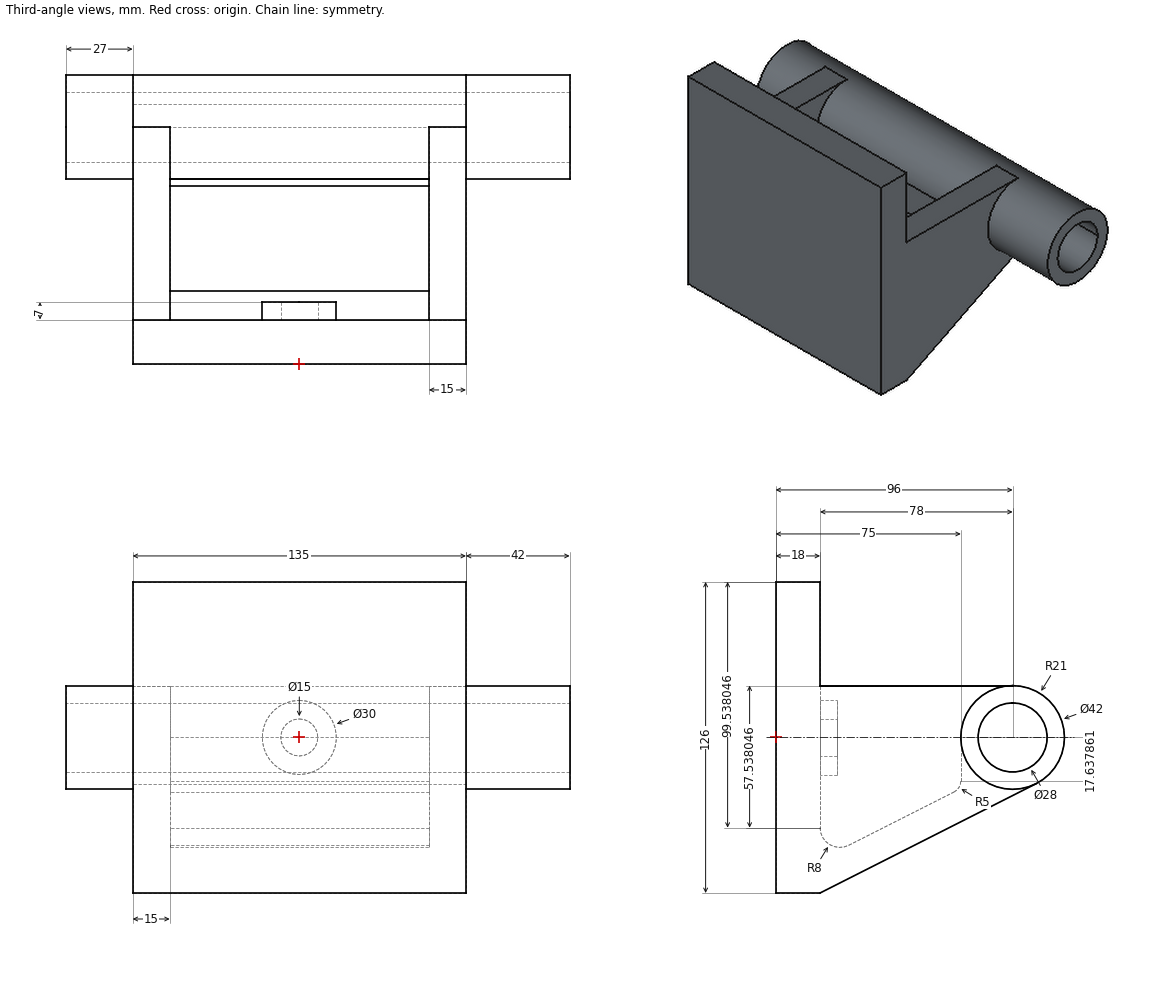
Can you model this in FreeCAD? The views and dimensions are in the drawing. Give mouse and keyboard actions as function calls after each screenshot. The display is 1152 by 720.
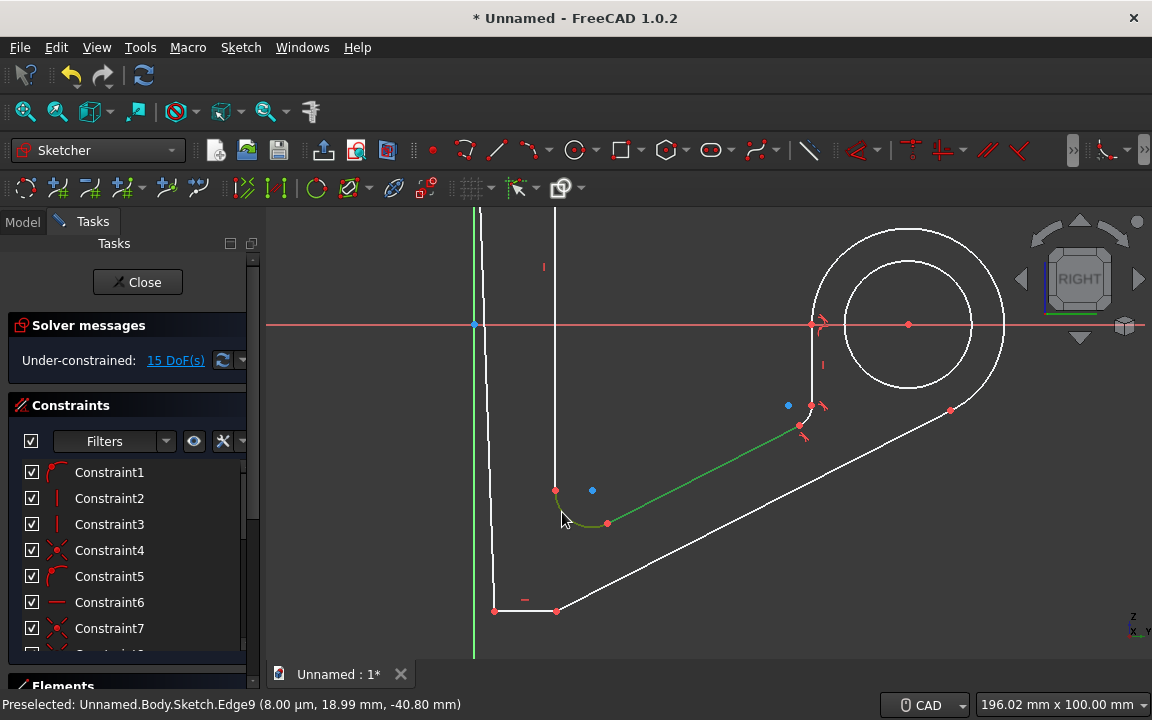
key(t)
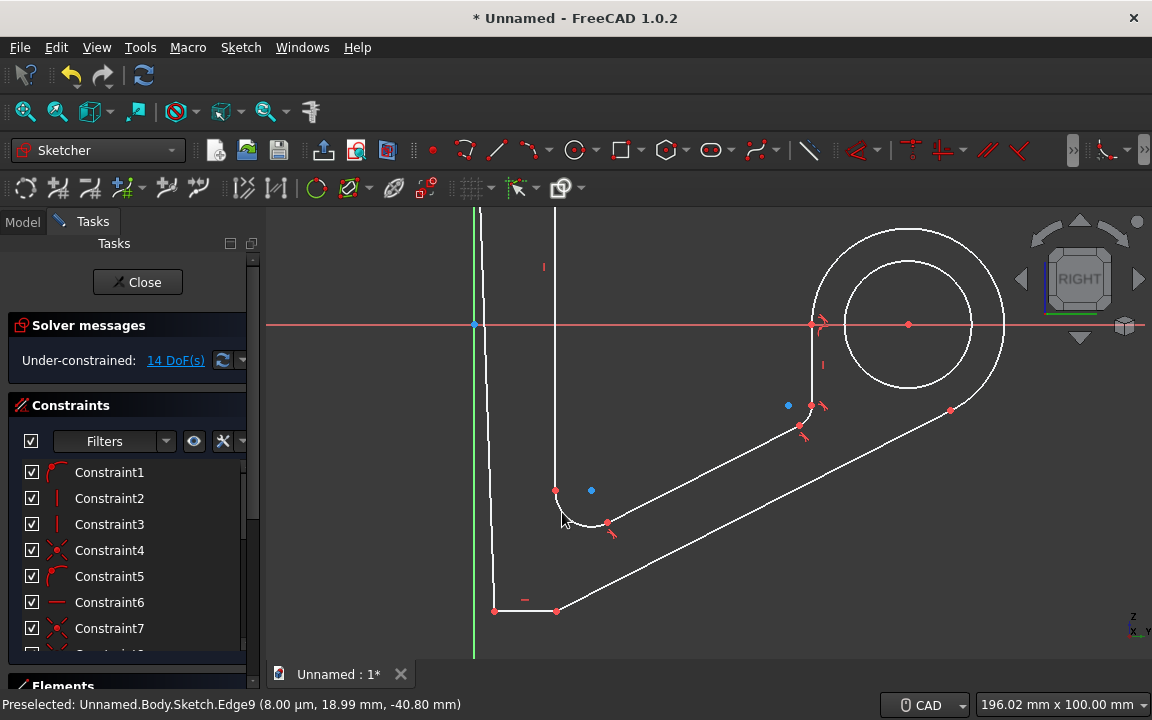
click(555, 356)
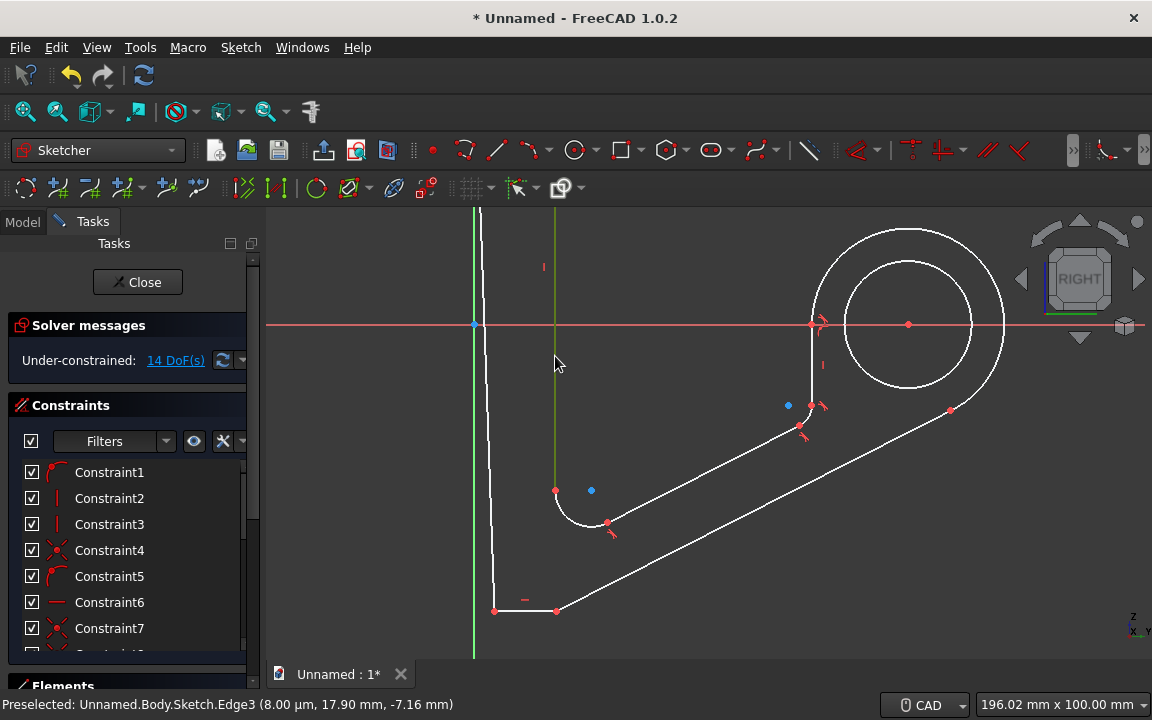
click(562, 511)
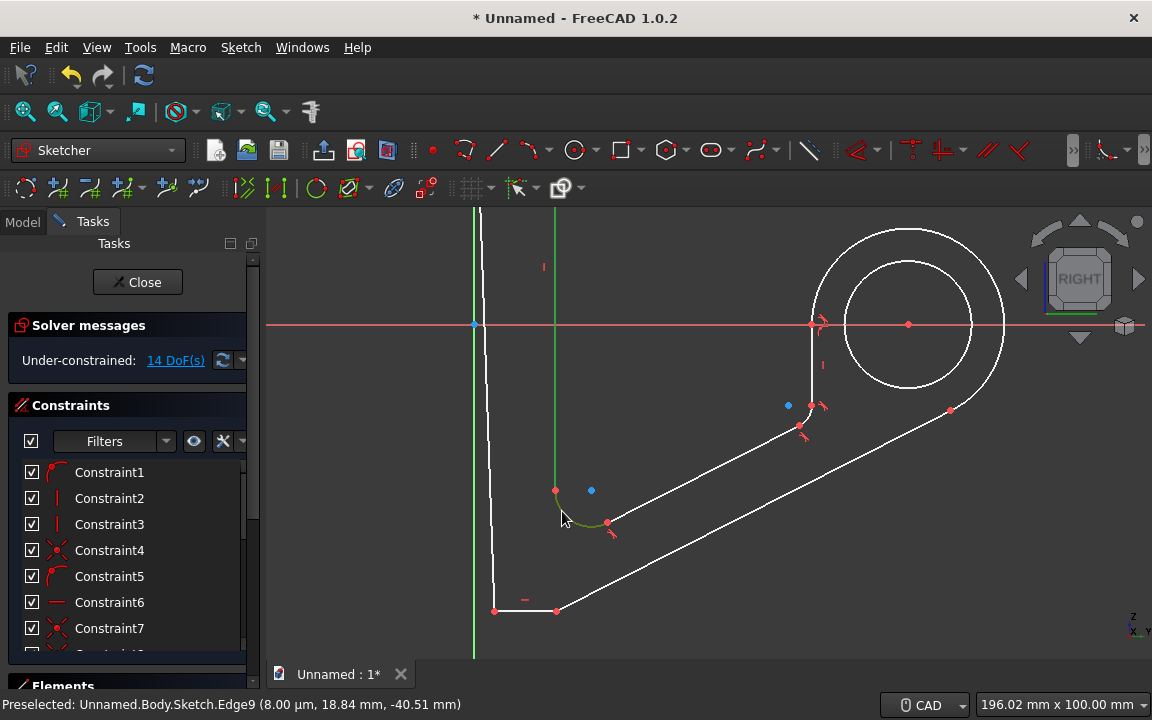
key(t)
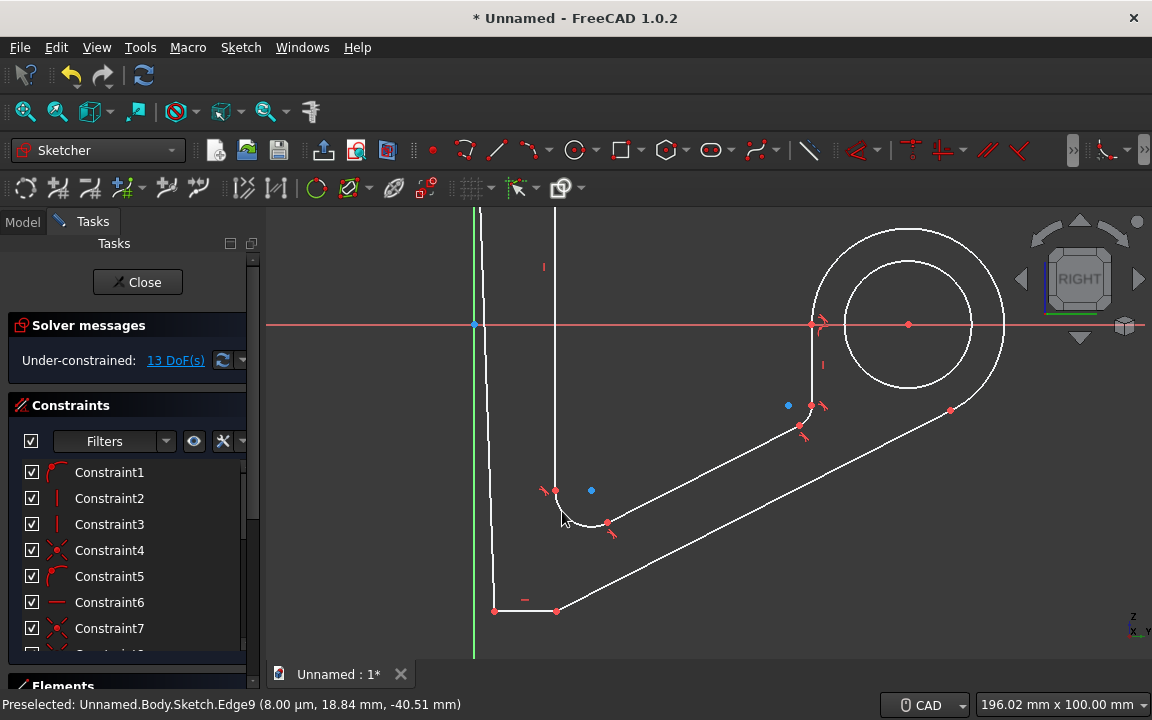
click(675, 551)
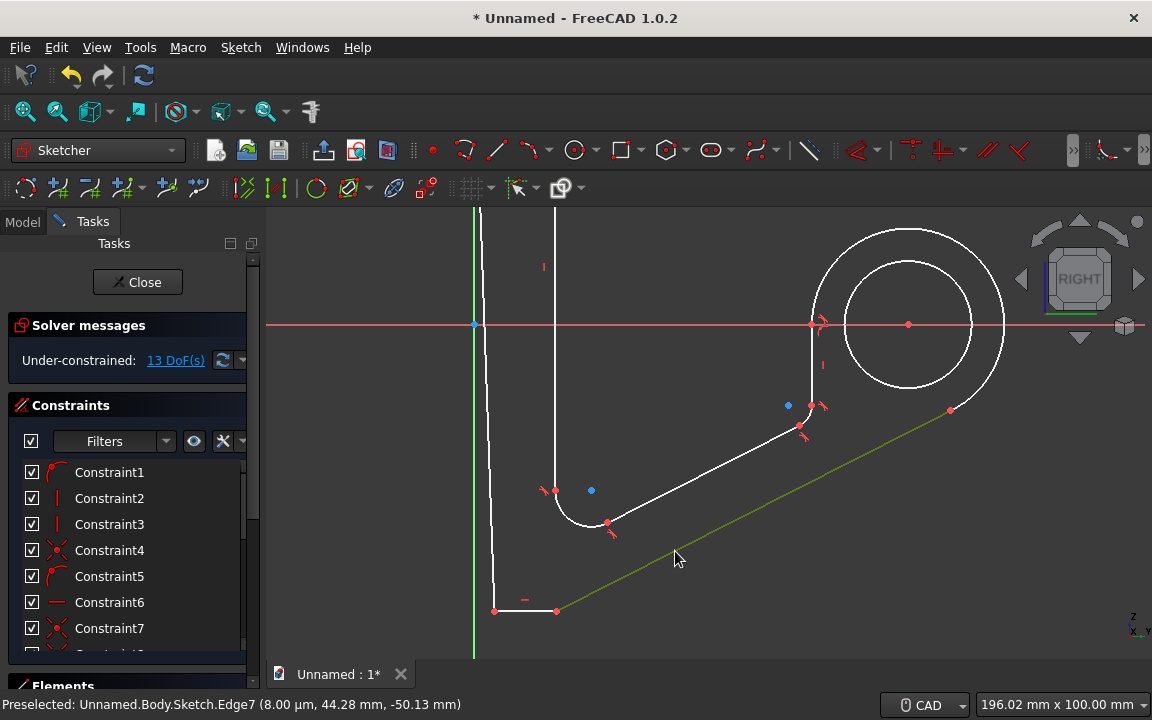
click(959, 243)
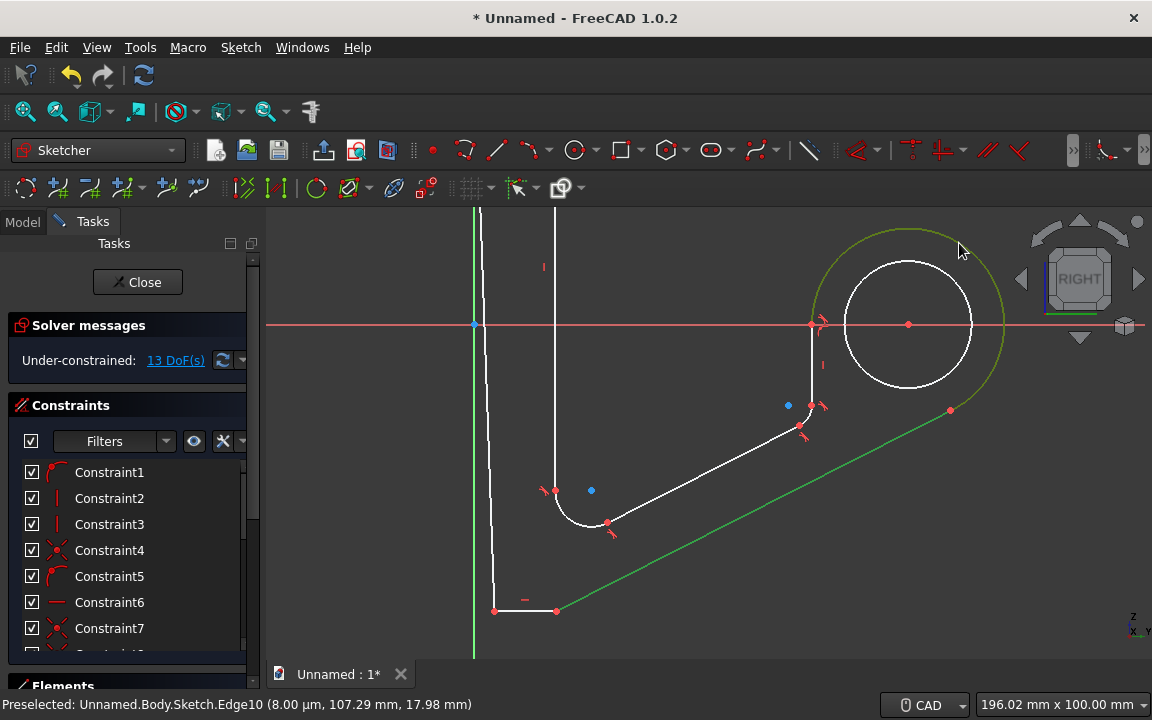
key(t)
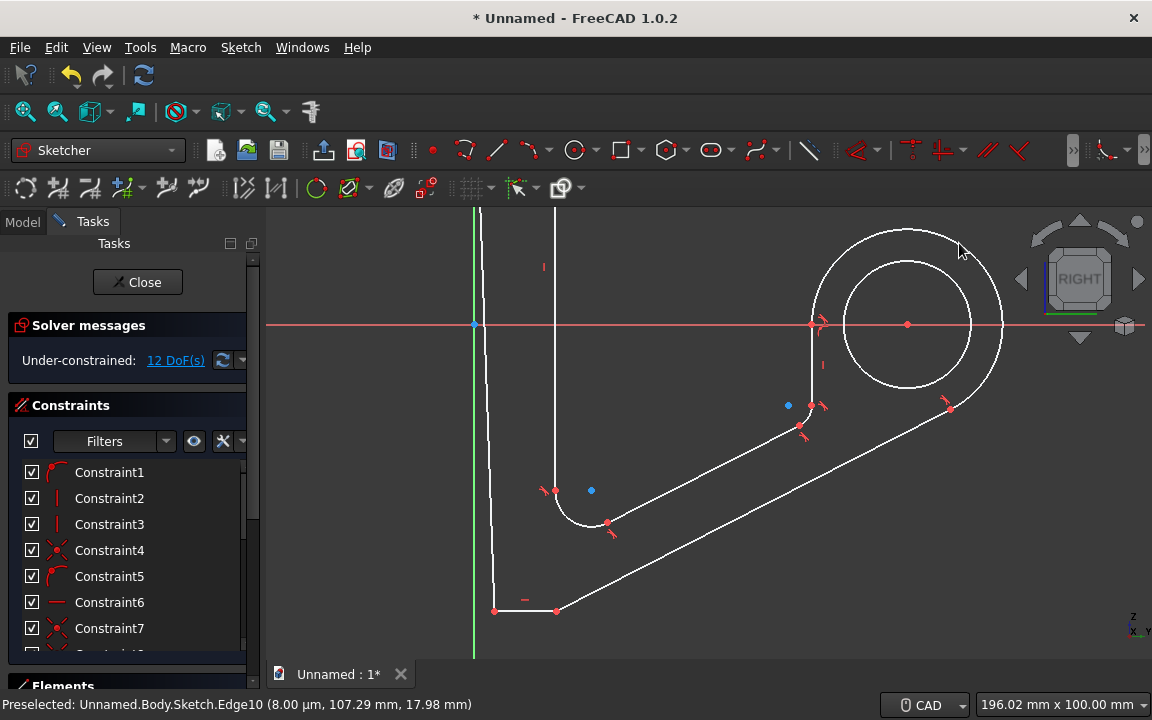
click(488, 440)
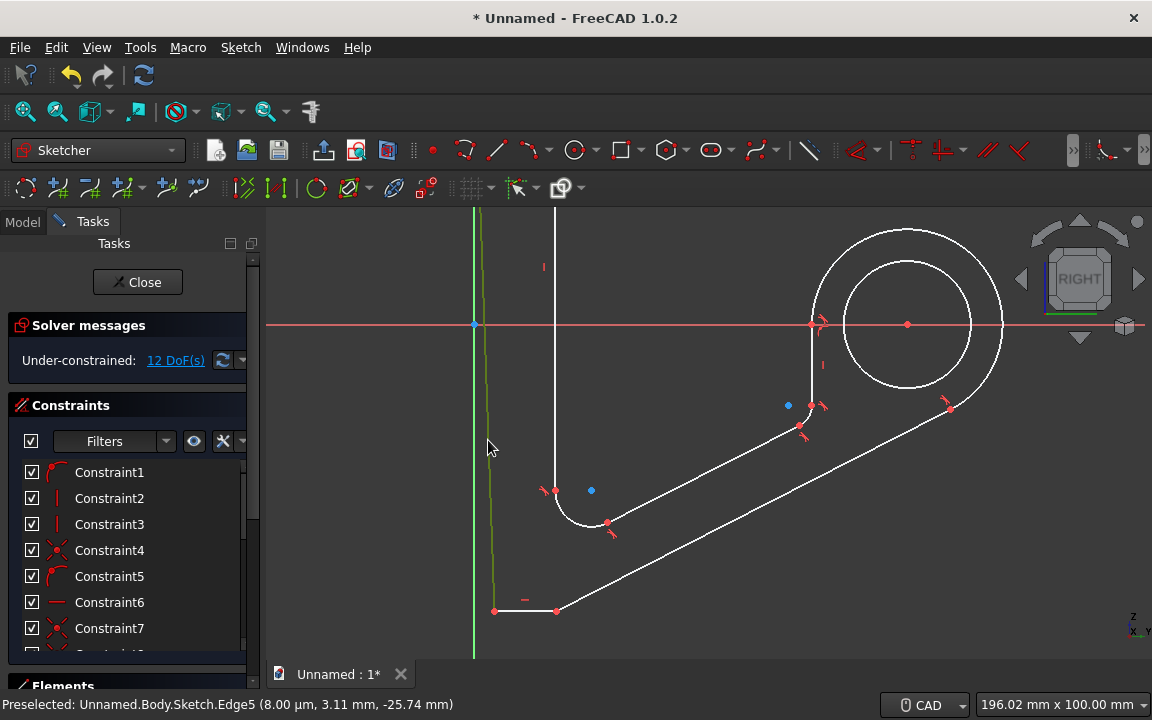
key(v)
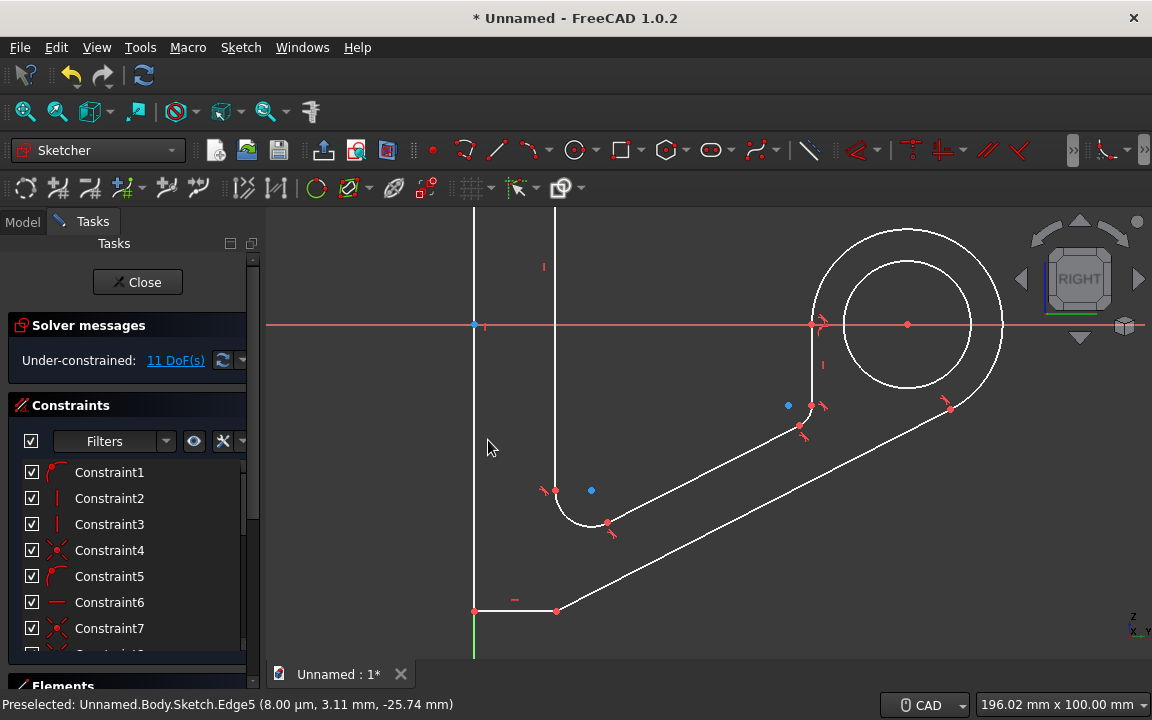
scroll(573, 521, down, 4)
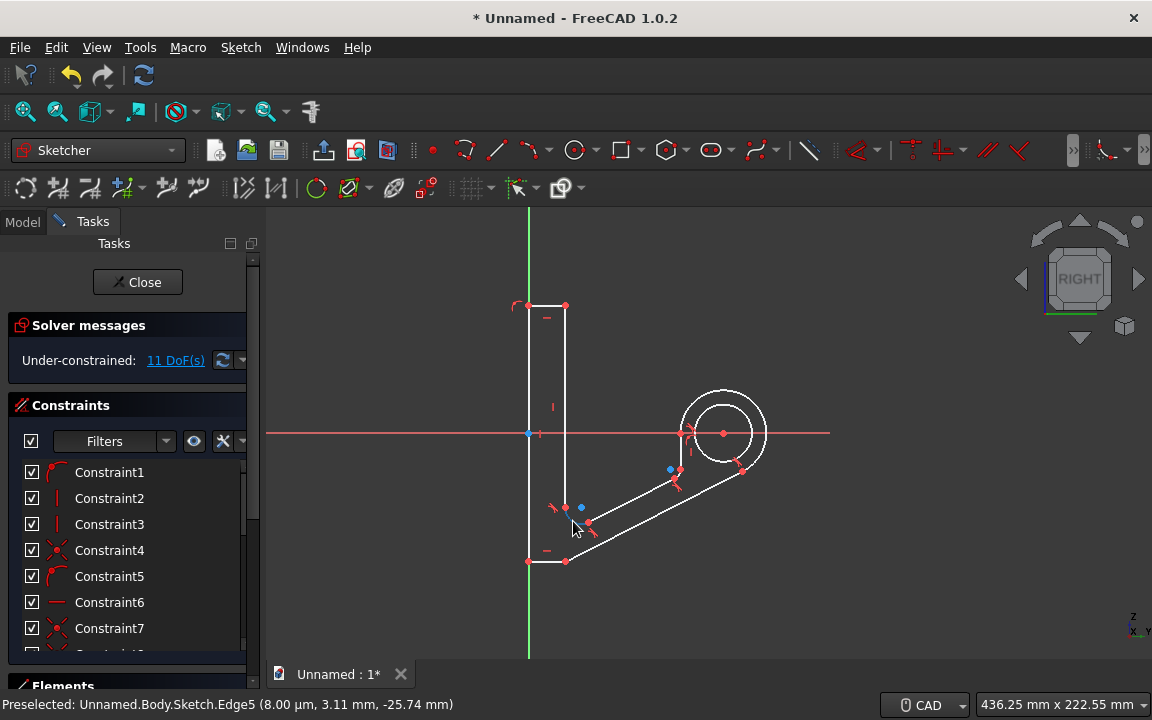
click(565, 306)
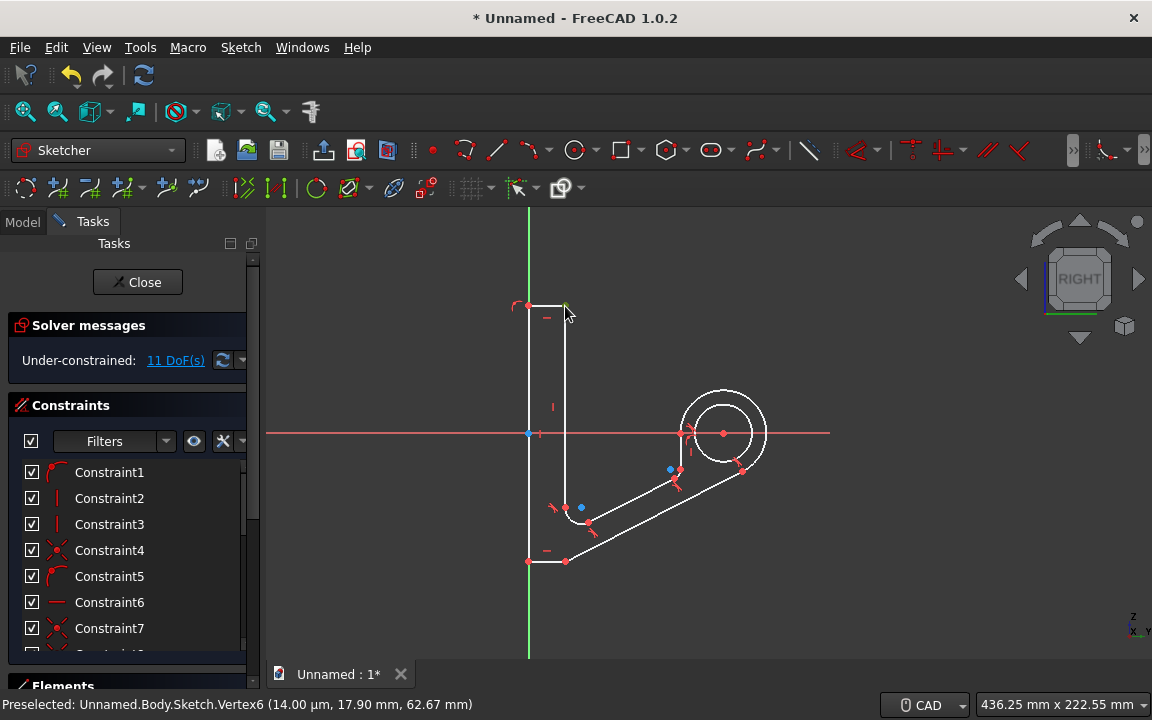
click(566, 562)